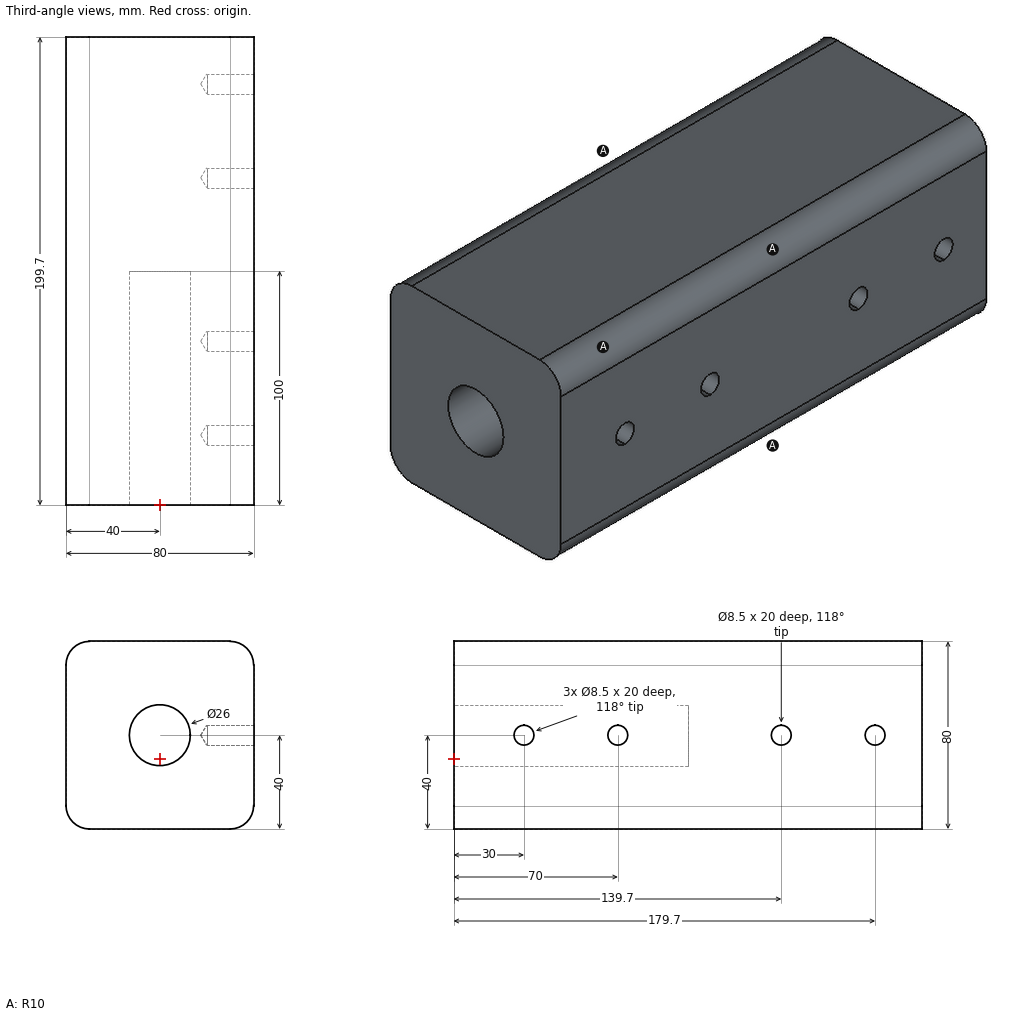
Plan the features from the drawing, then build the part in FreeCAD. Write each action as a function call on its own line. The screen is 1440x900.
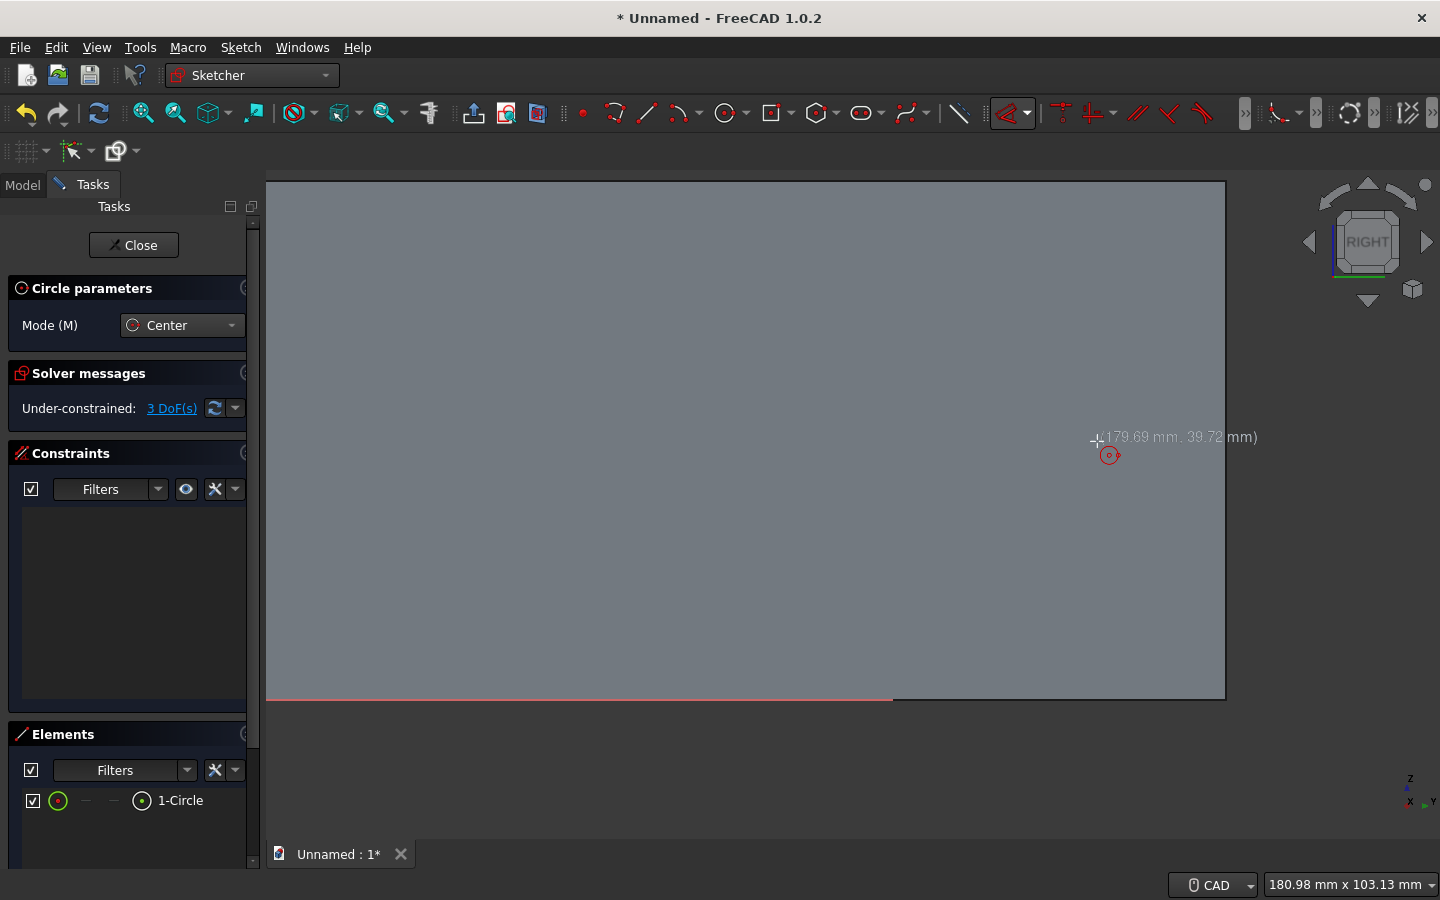
click(1096, 441)
click(1116, 421)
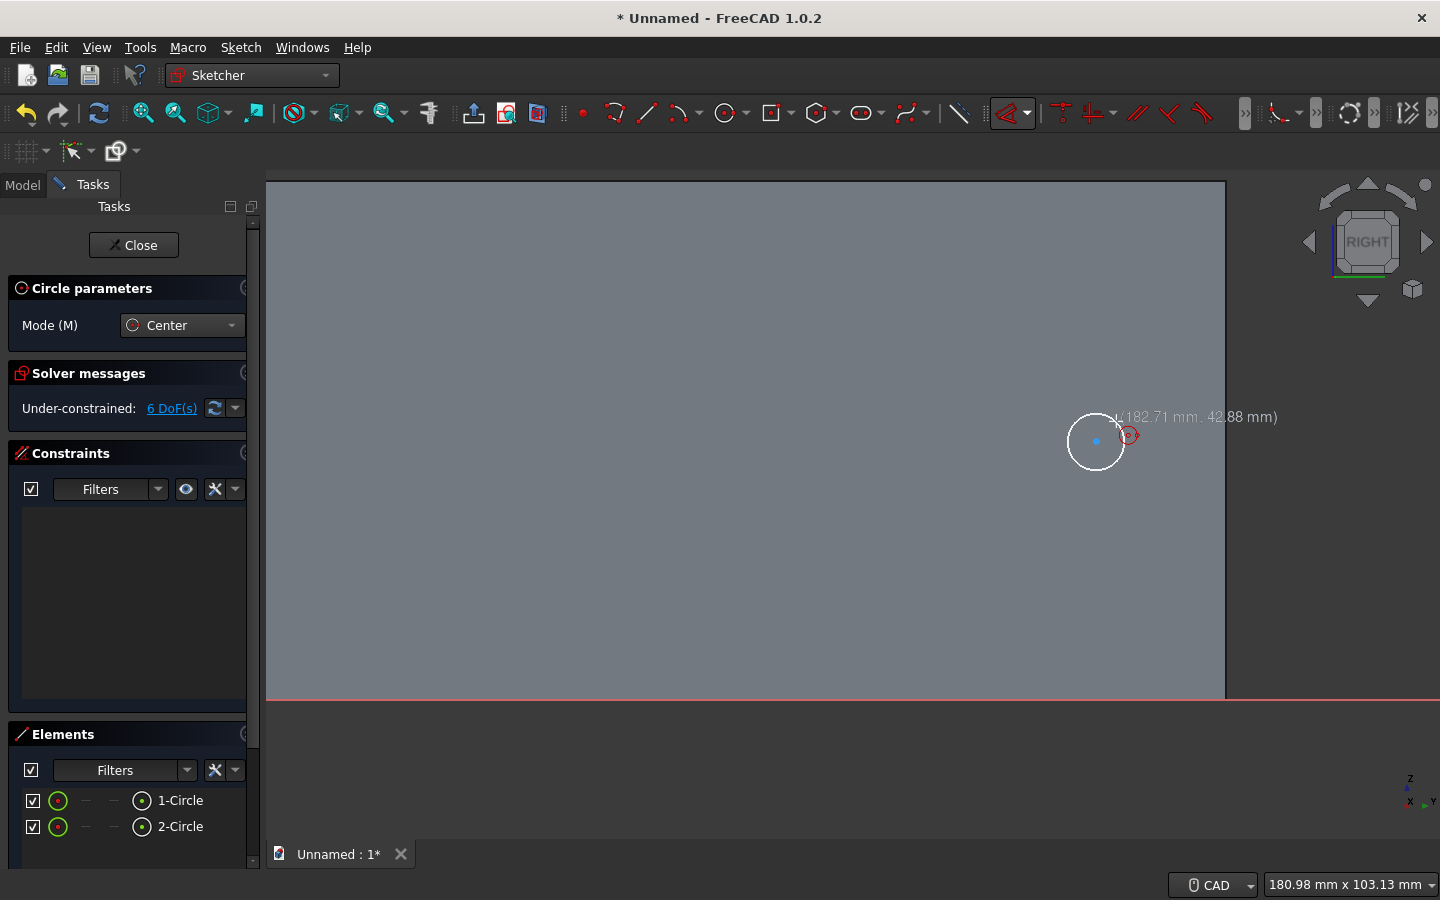
click(385, 441)
click(404, 421)
key(Escape)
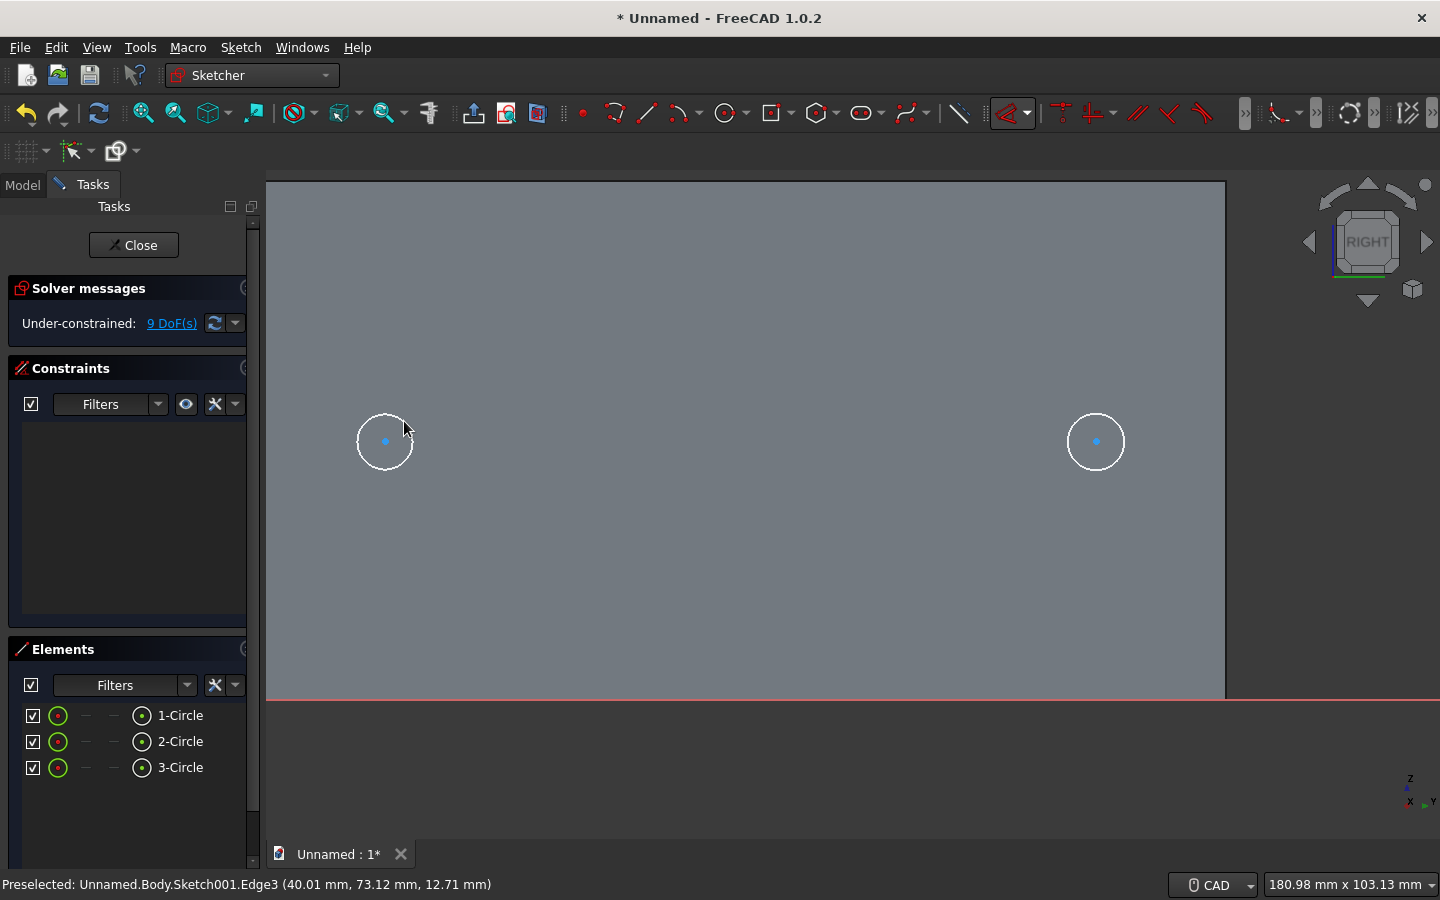
scroll(1097, 441, down, 3)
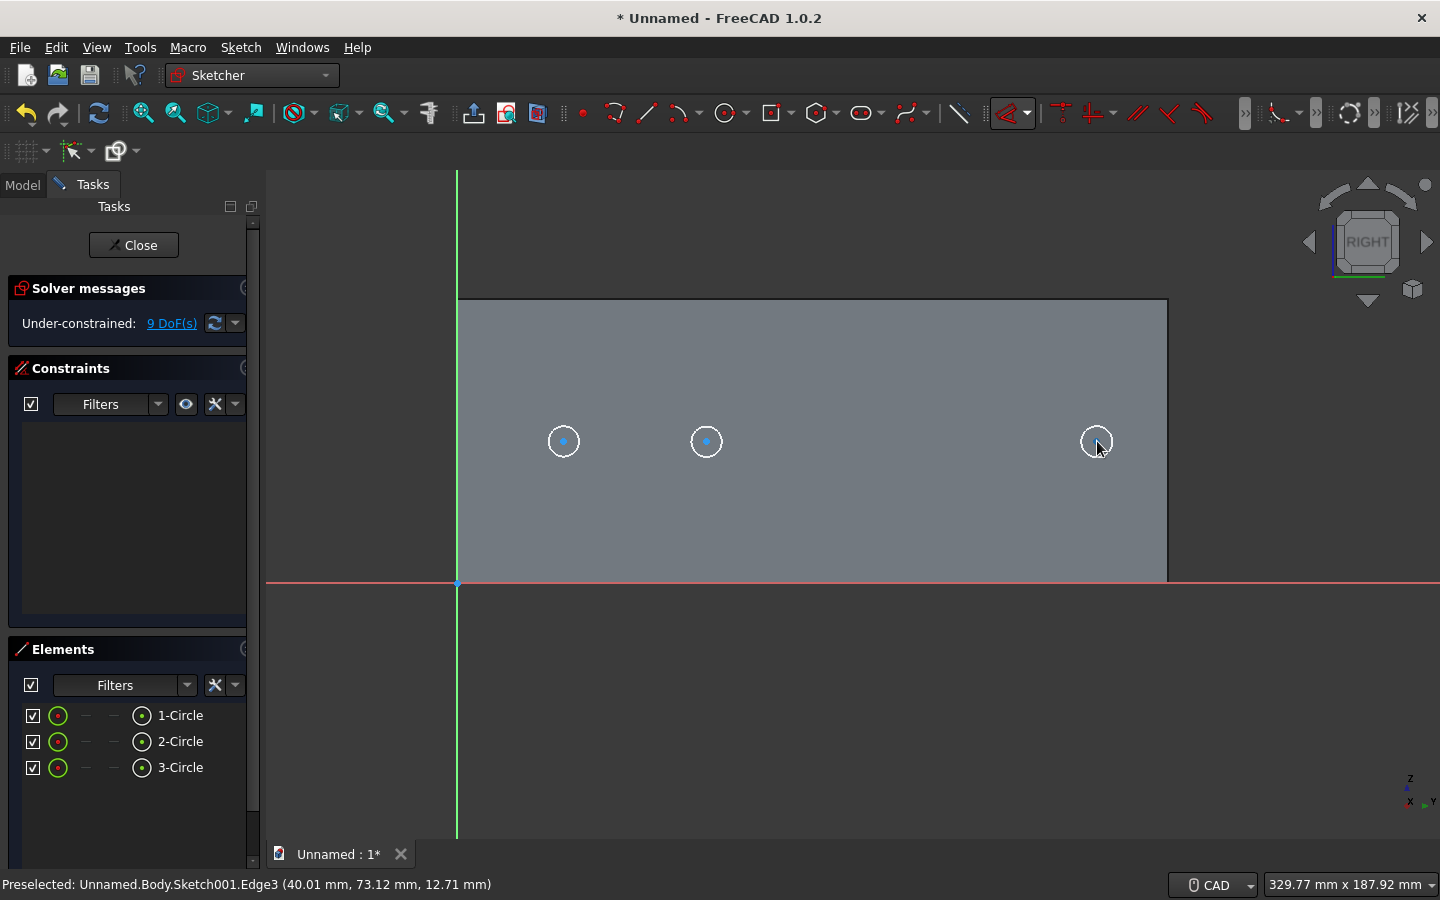
click(574, 431)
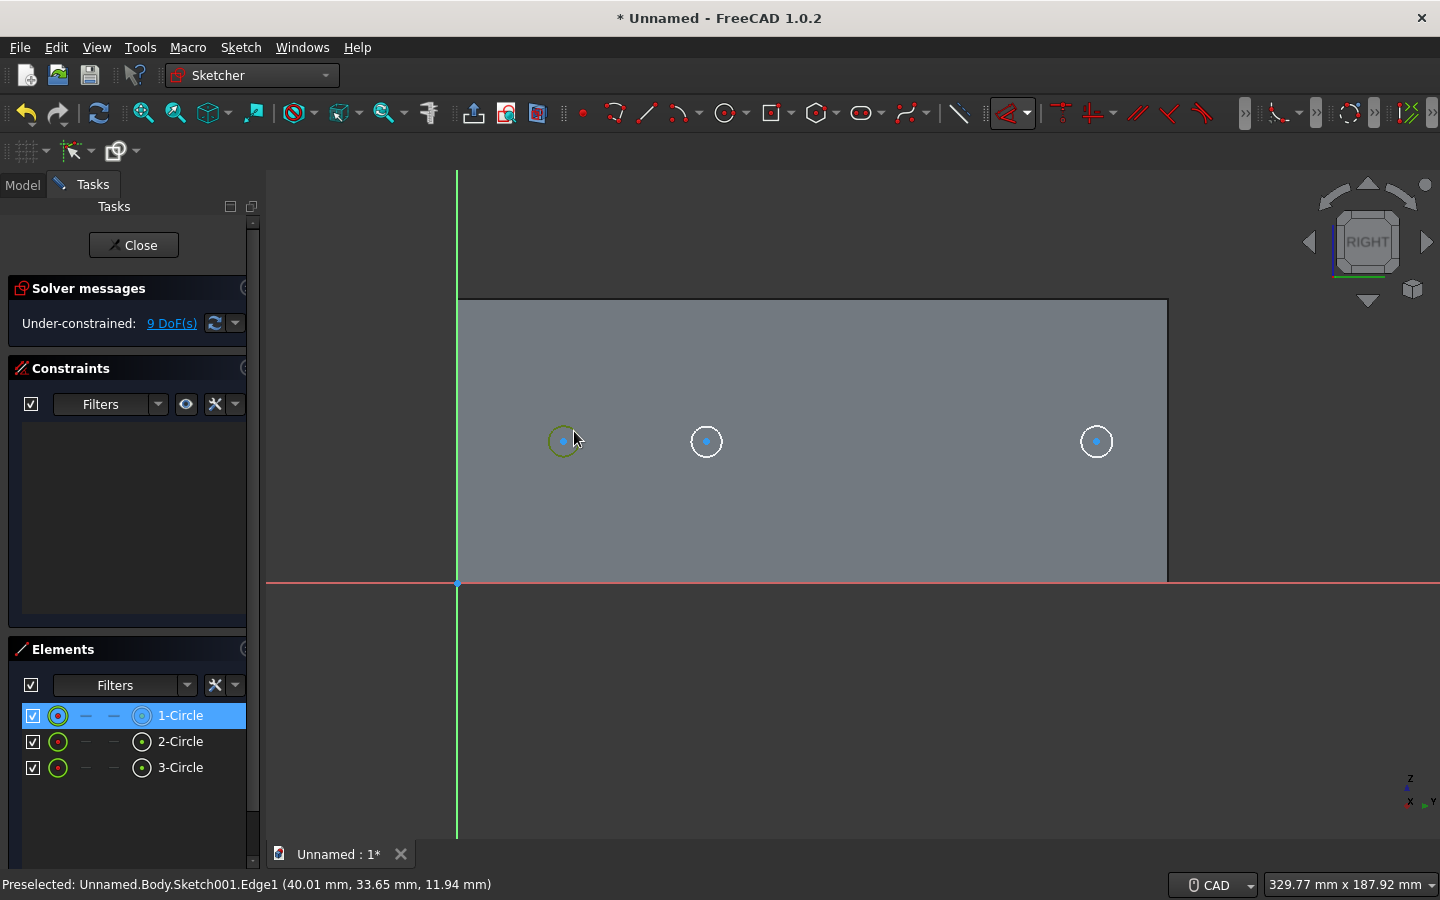
click(1108, 431)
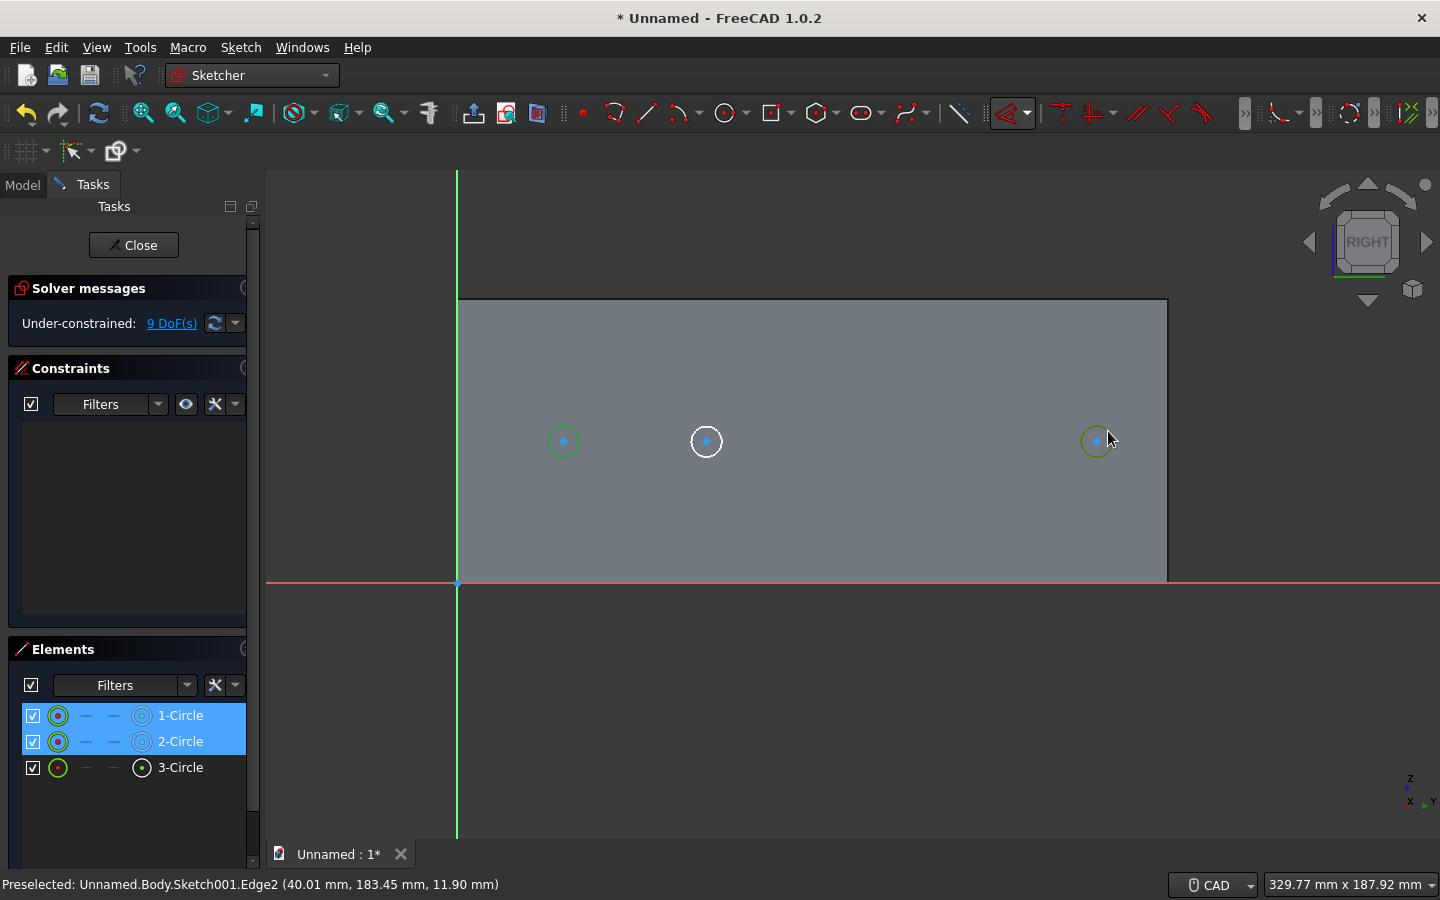
click(717, 431)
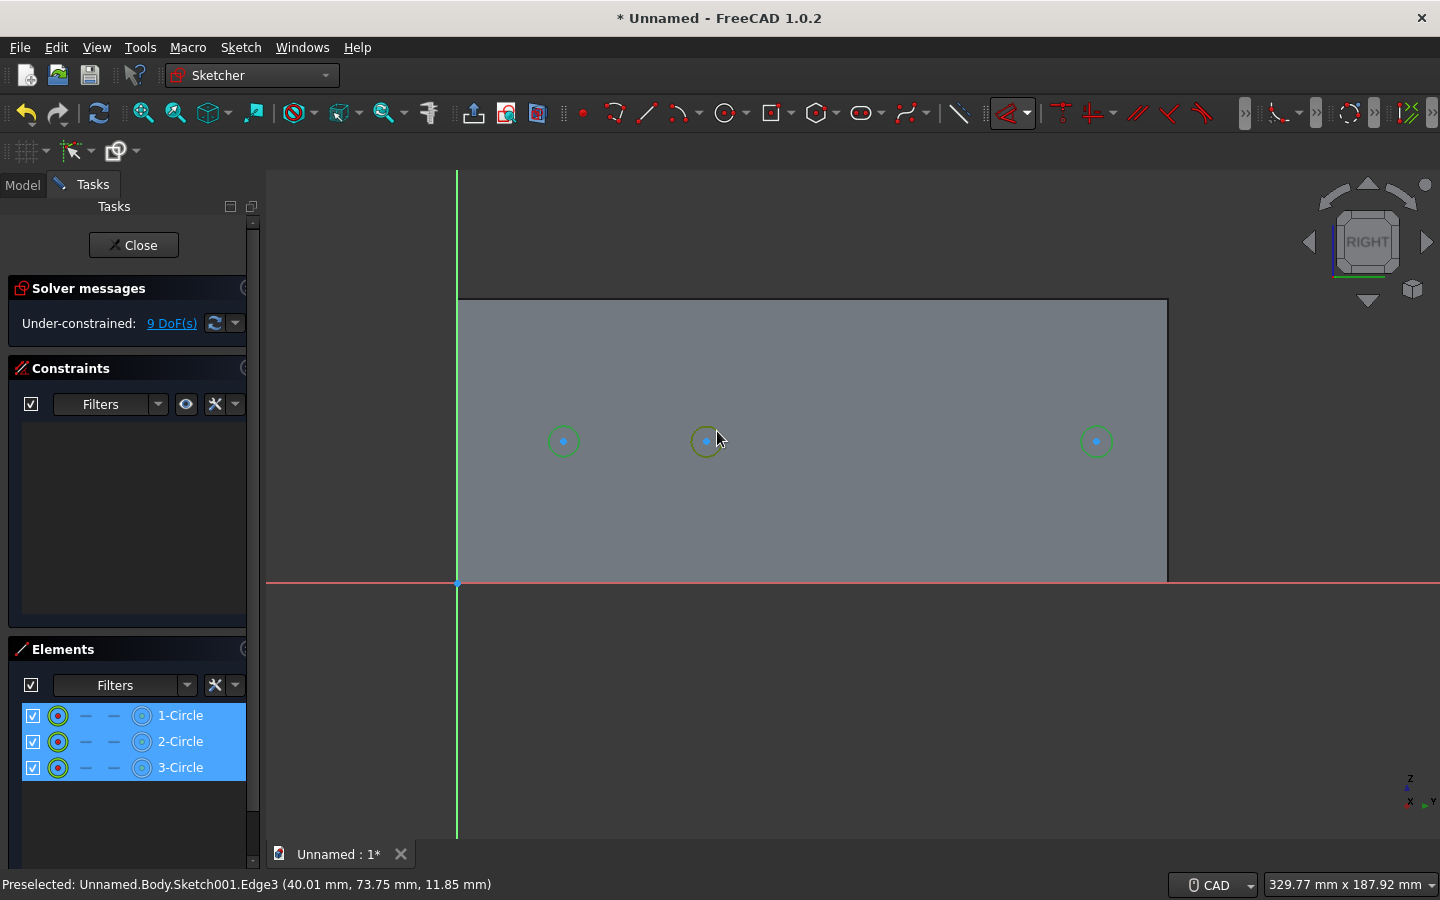
key(e)